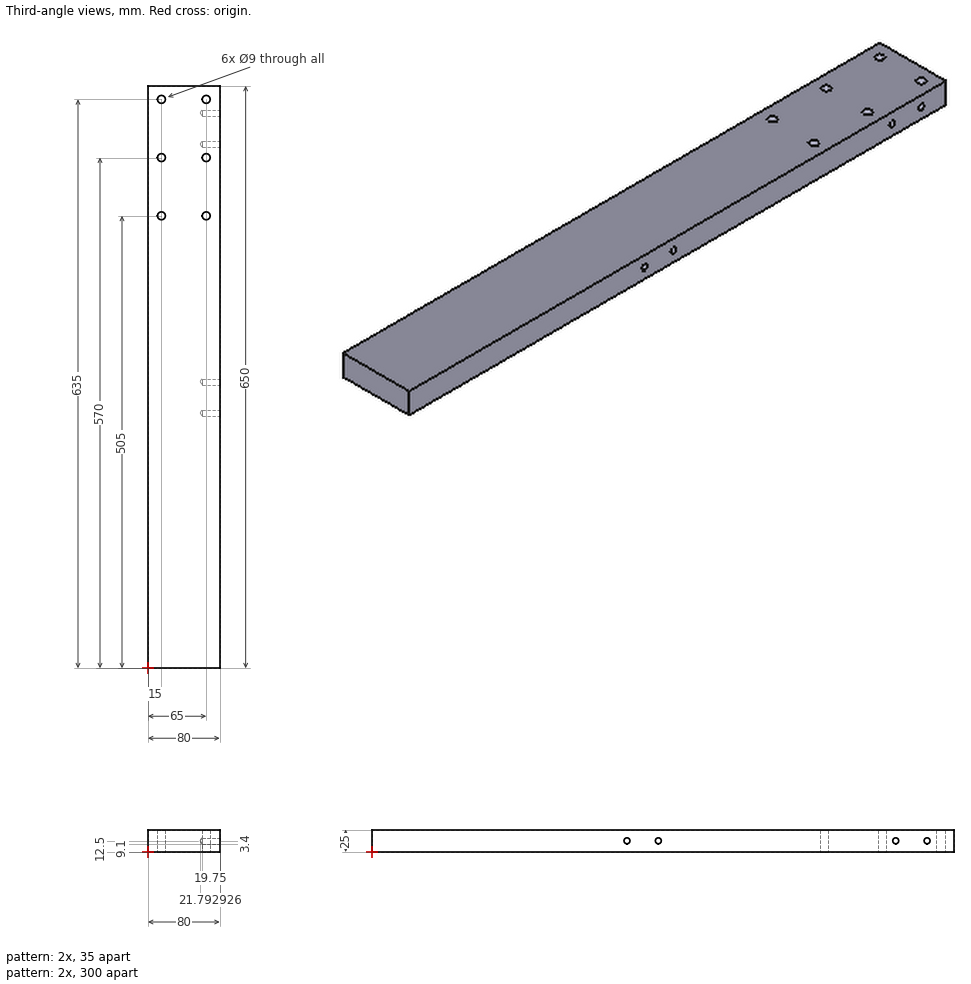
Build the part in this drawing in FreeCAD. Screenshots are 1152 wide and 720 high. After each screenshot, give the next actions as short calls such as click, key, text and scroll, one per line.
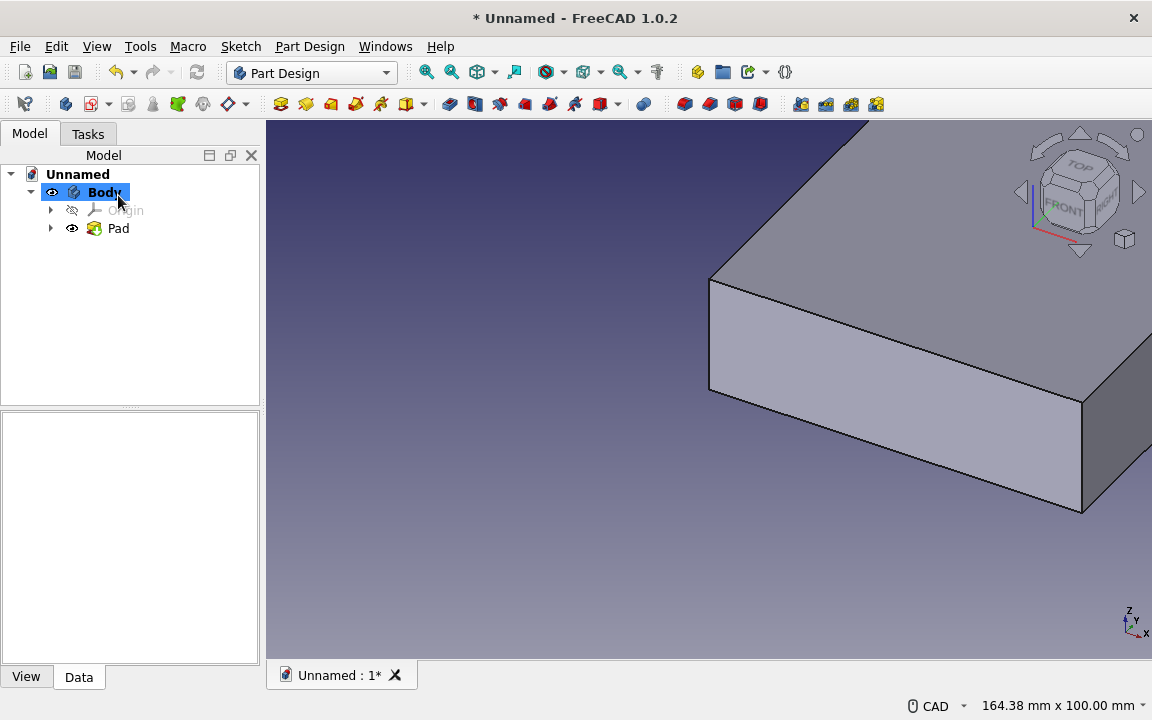
click(427, 72)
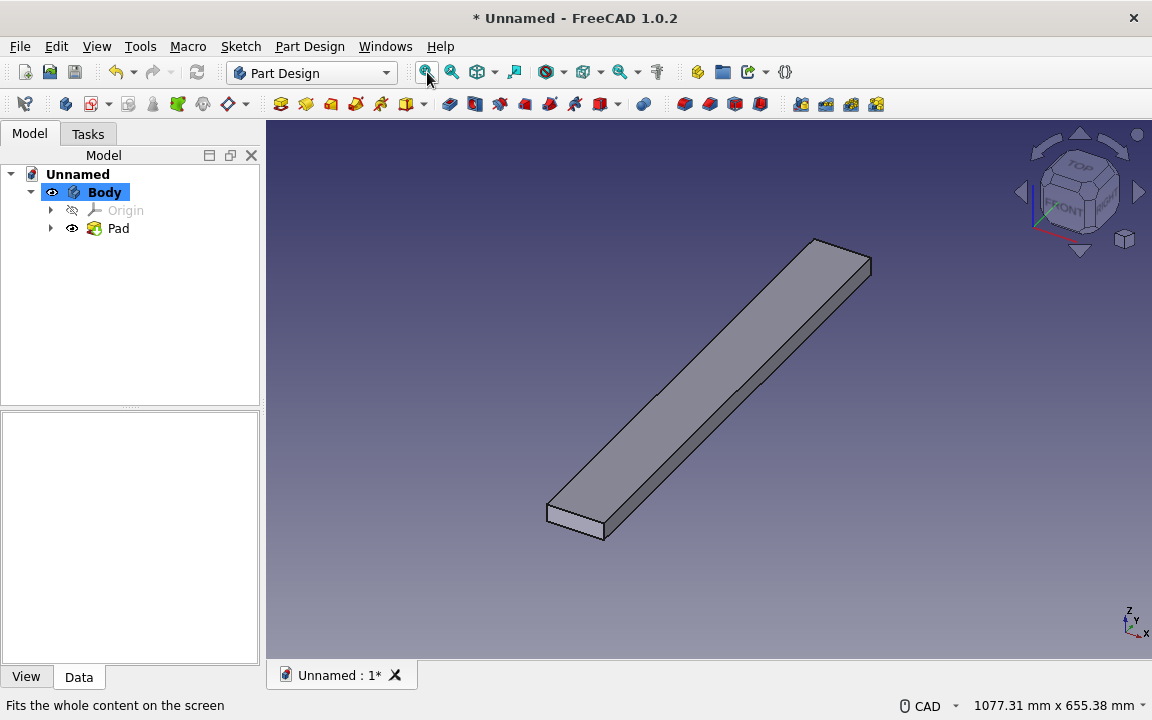
click(824, 266)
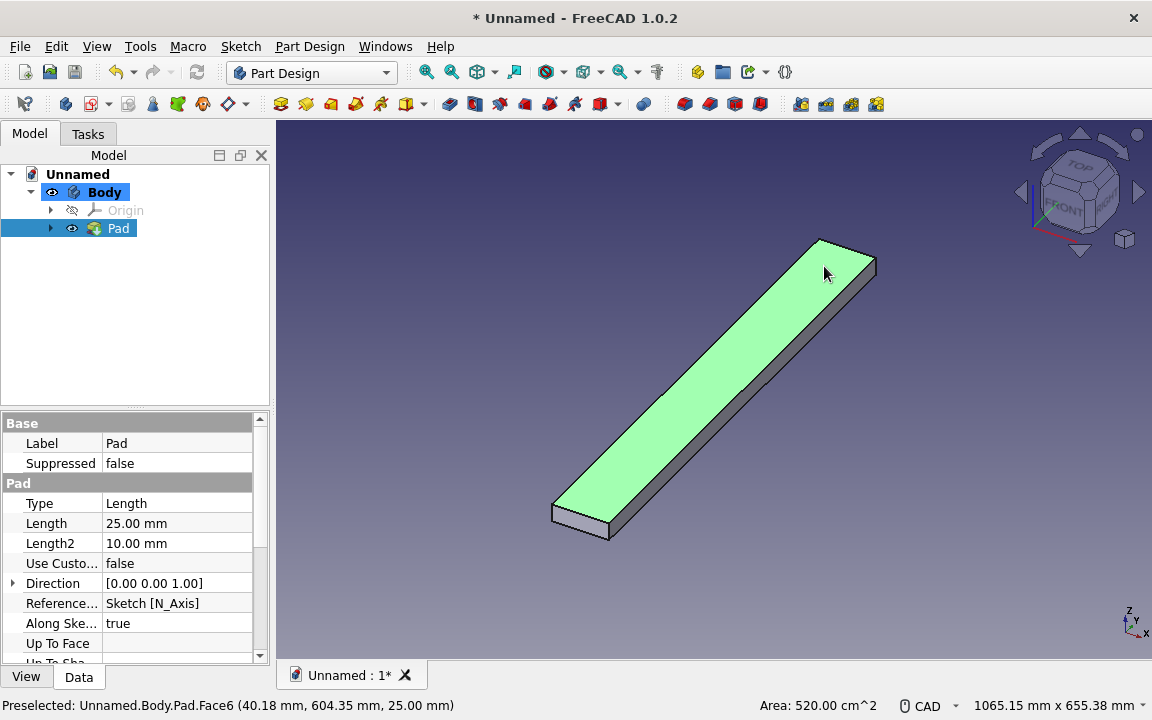
click(90, 104)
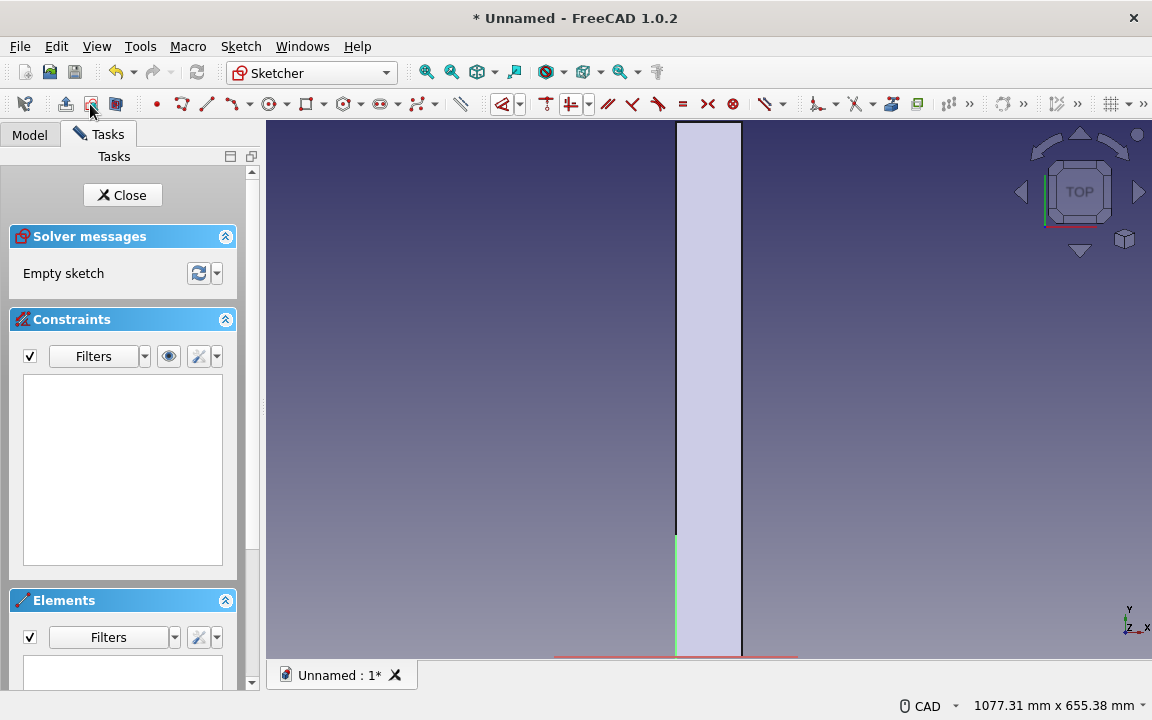
scroll(640, 390, down, 5)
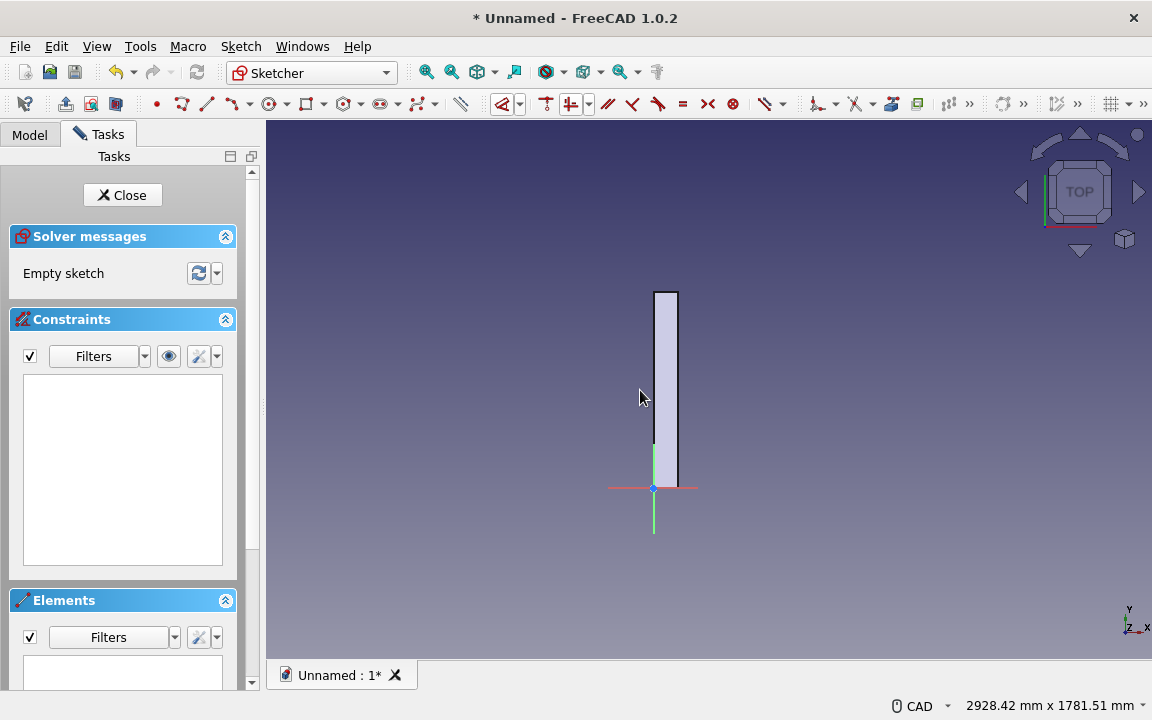
scroll(670, 305, up, 10)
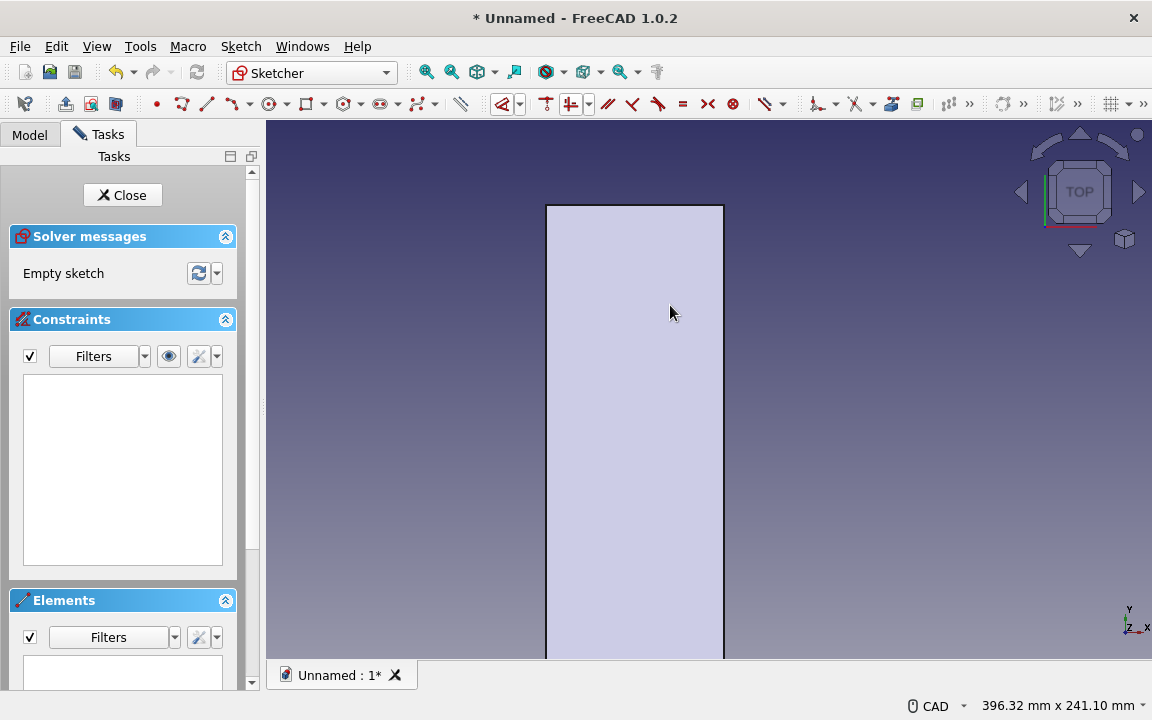
click(268, 104)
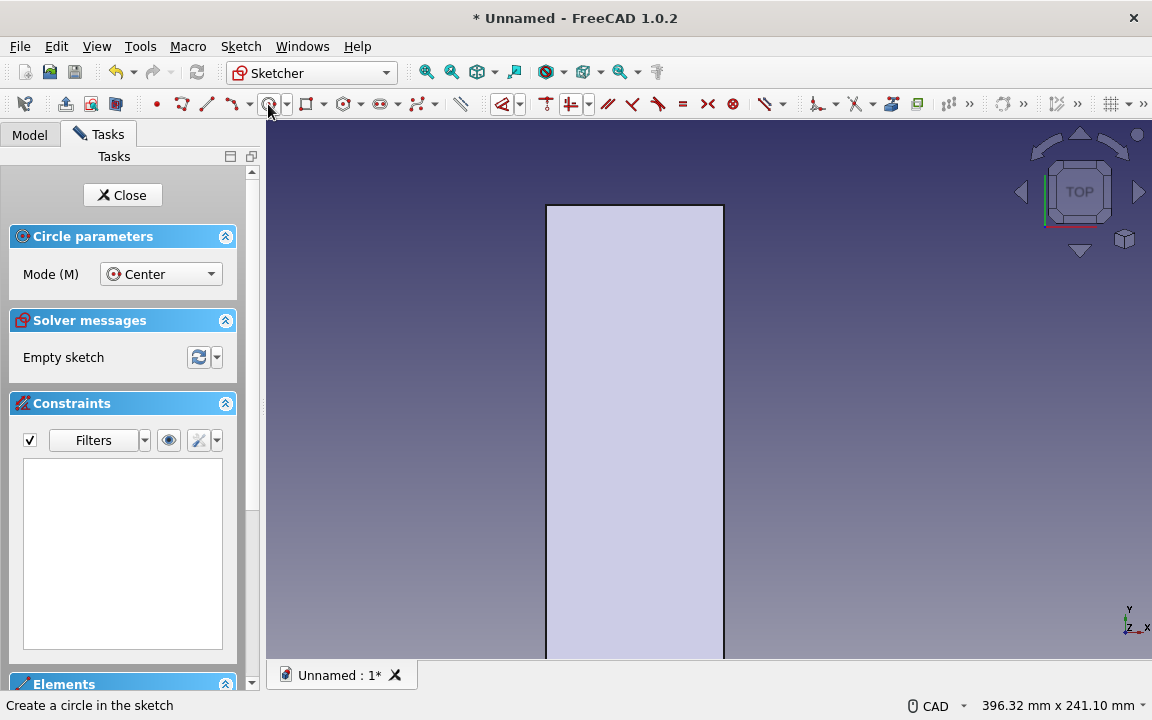
scroll(579, 239, up, 5)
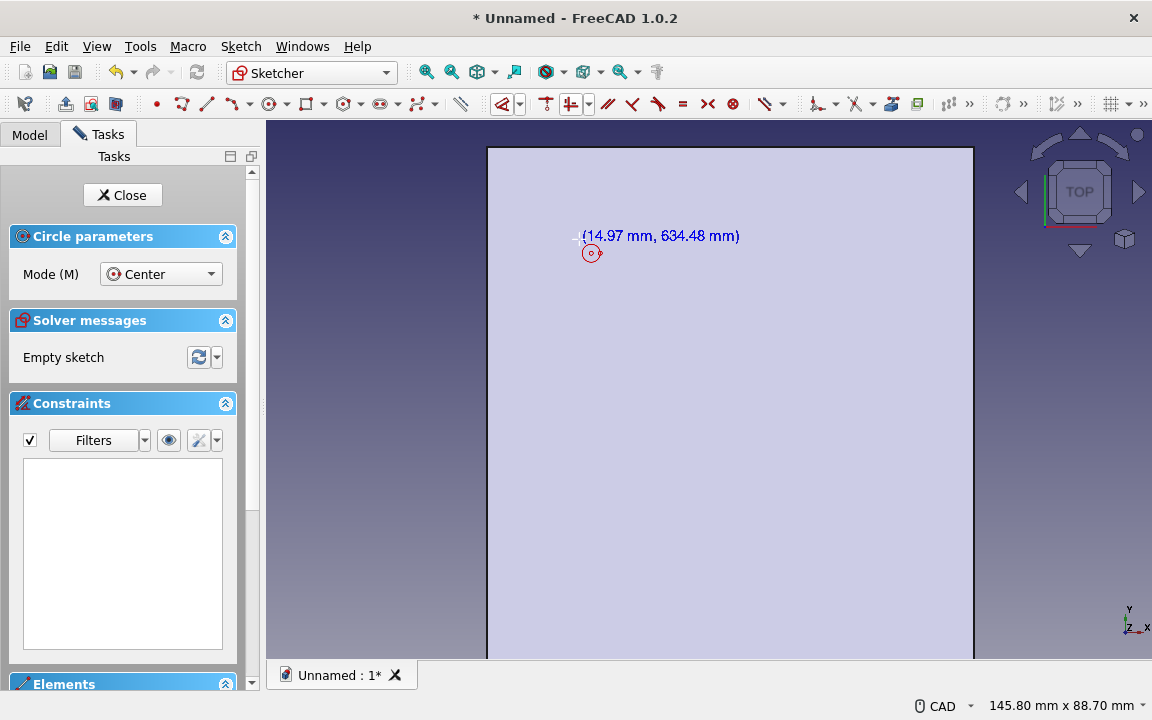
click(579, 238)
move(598, 219)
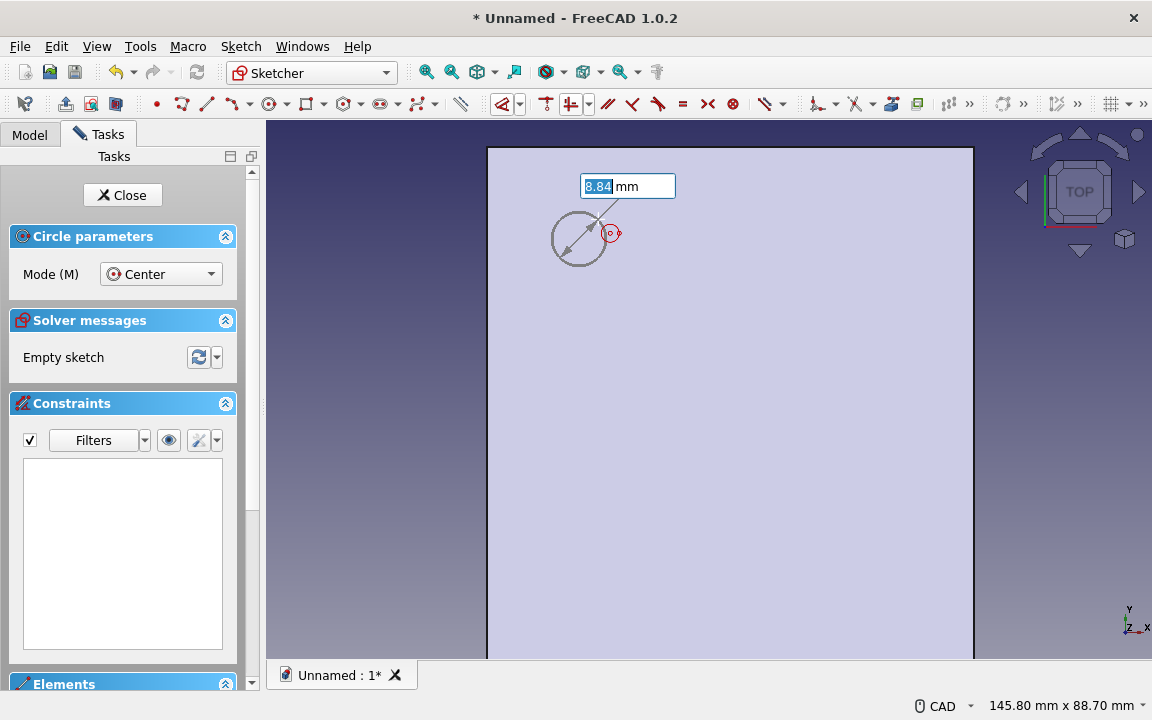
text(9)
key(Return)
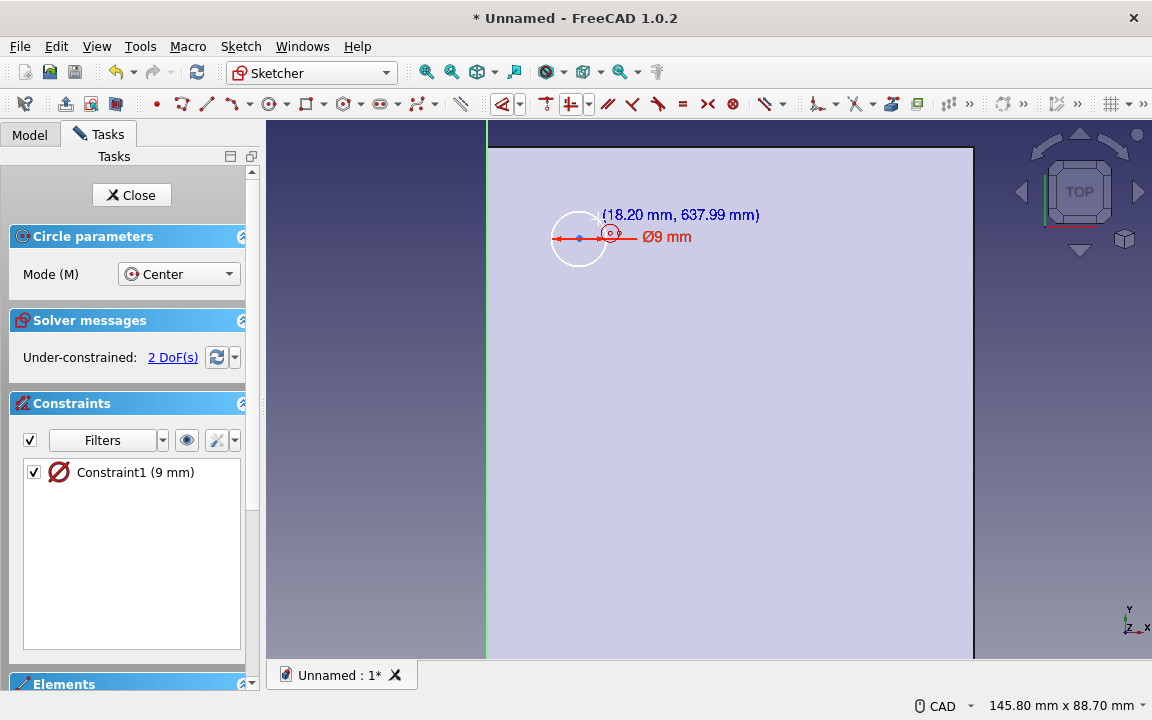
click(882, 238)
move(902, 219)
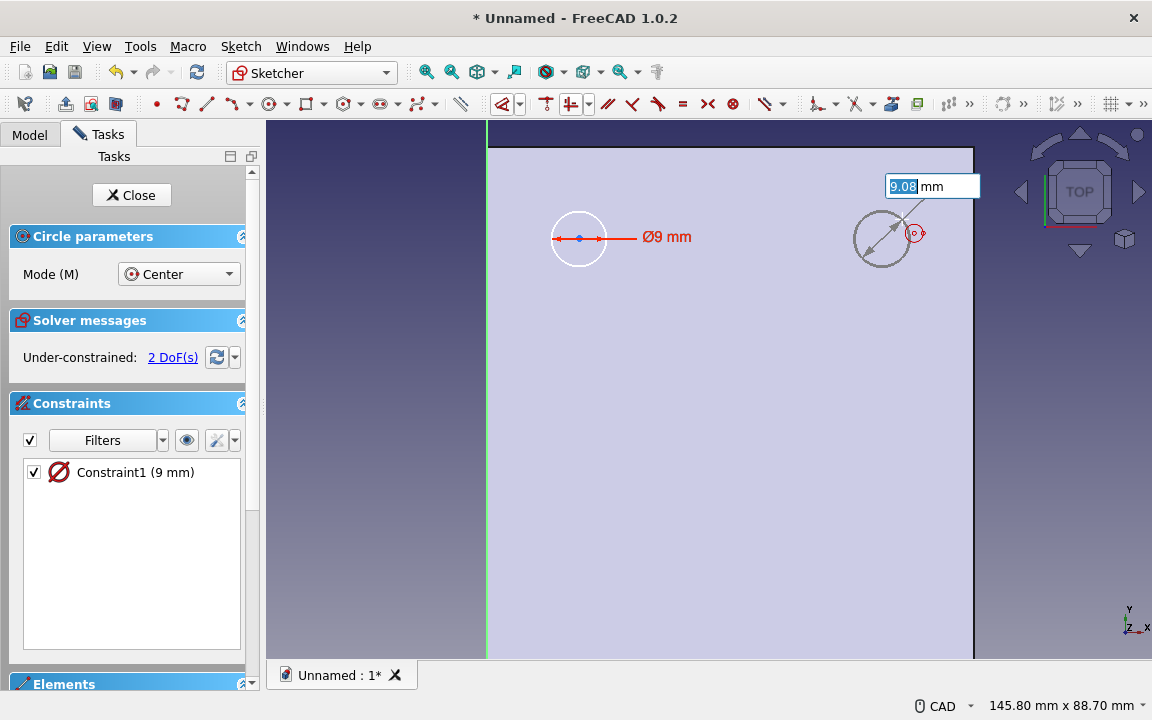
text(9)
key(Return)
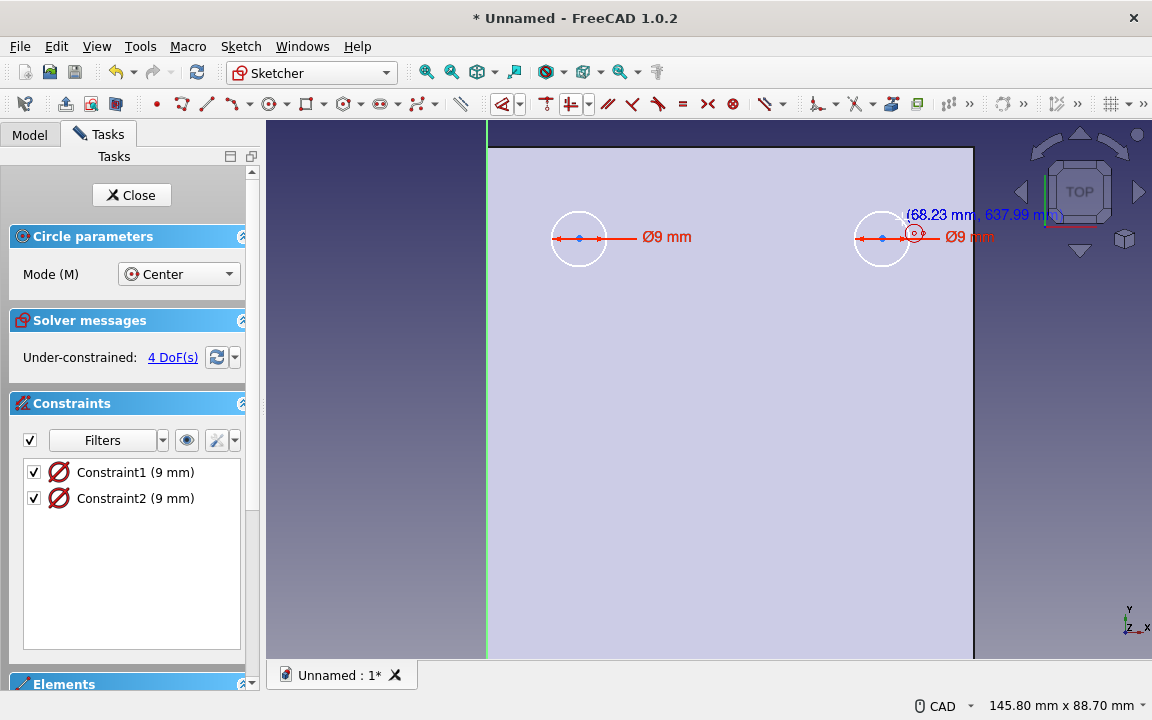
scroll(588, 248, down, 5)